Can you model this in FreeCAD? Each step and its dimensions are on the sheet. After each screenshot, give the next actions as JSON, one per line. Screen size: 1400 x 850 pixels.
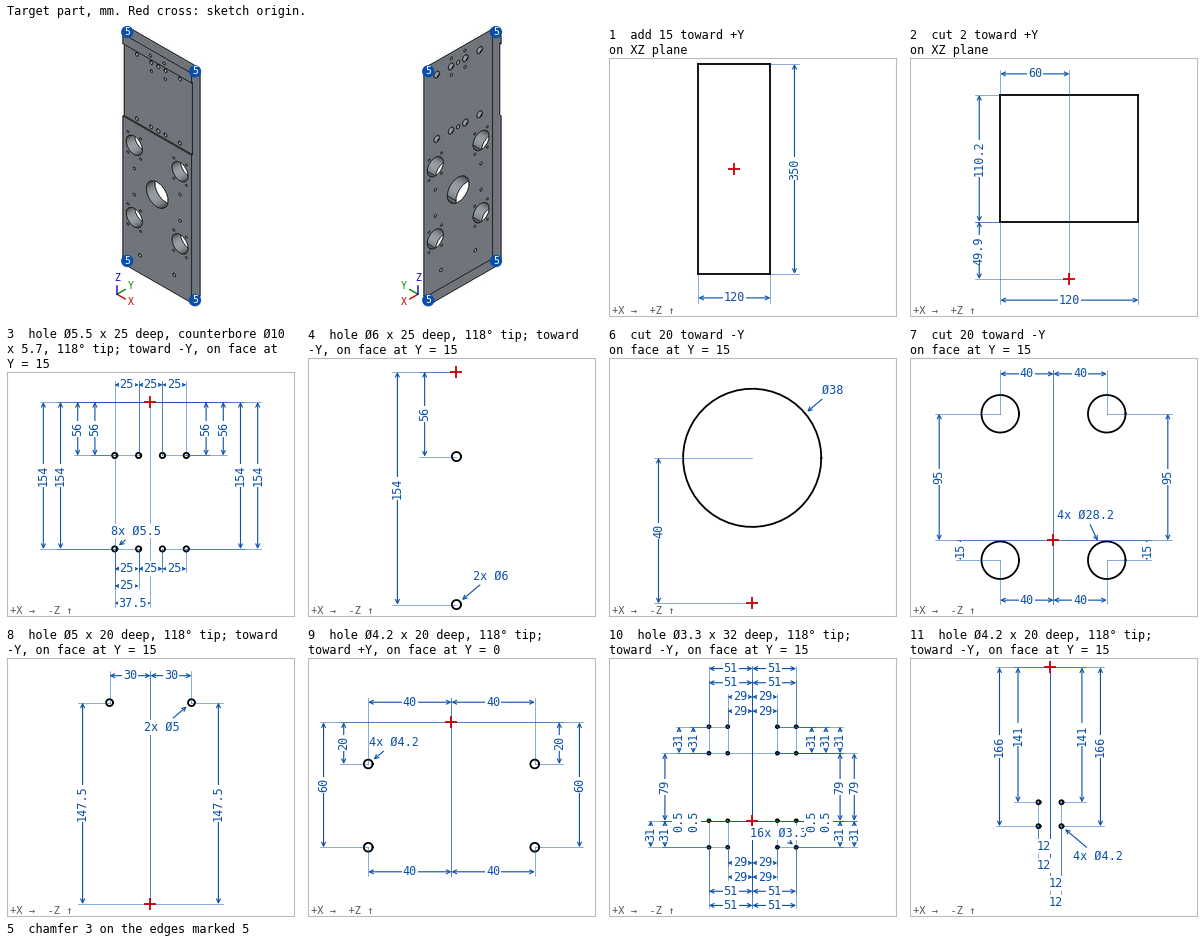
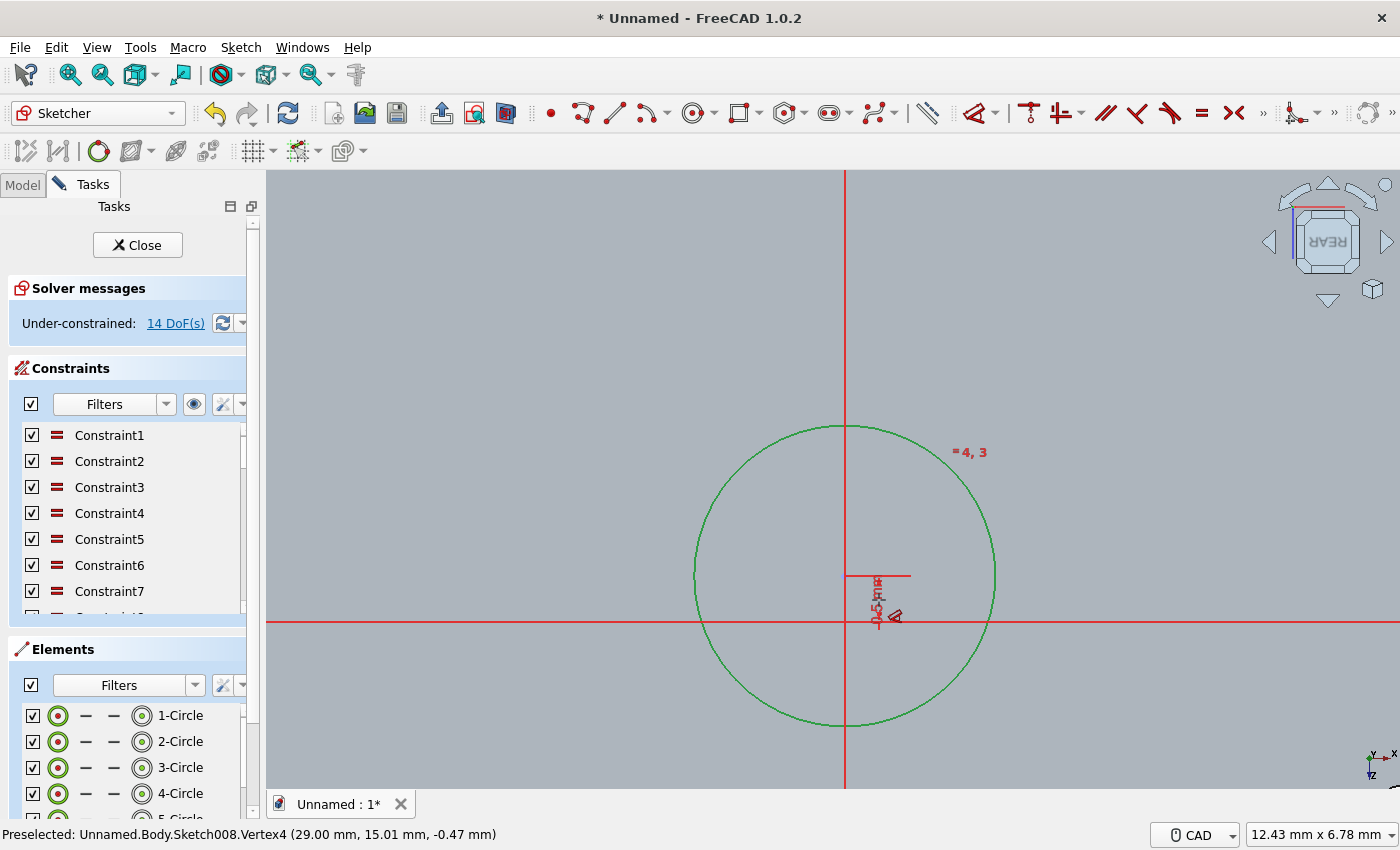
{"action": "scroll", "coordinate": [853, 601], "scroll_direction": "down", "scroll_amount": 17}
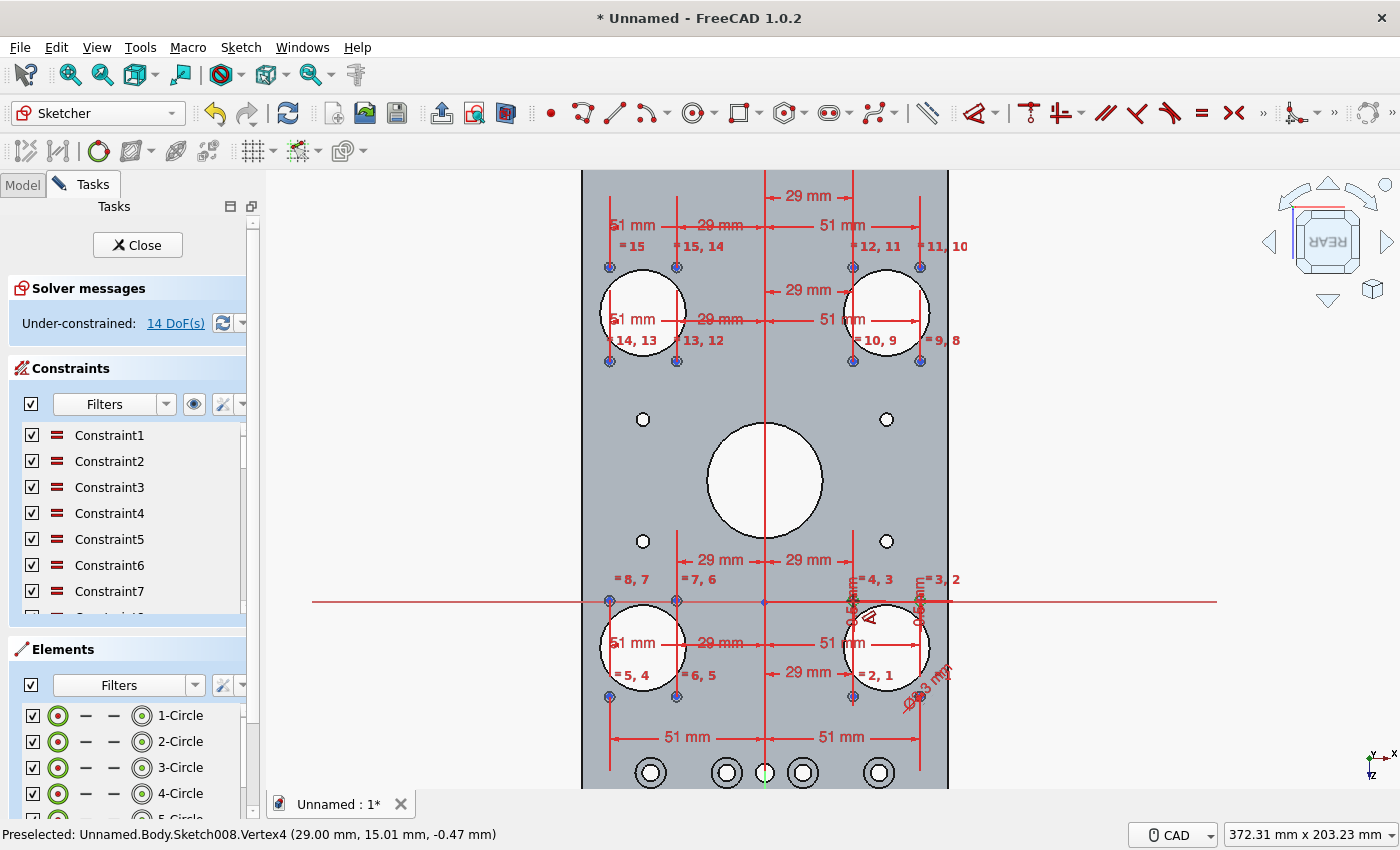
{"action": "scroll", "coordinate": [677, 601], "scroll_direction": "up", "scroll_amount": 17}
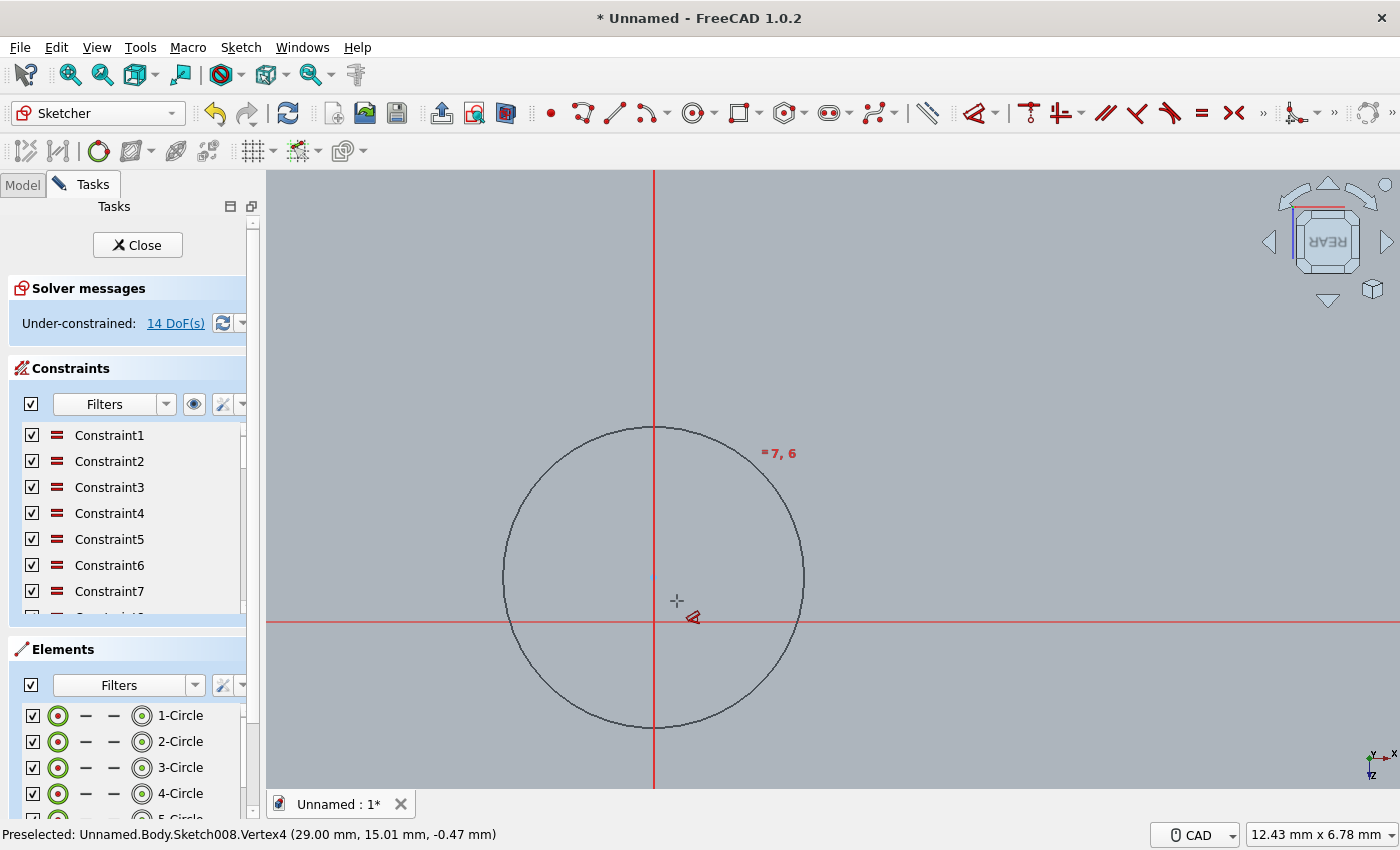
{"action": "left_click", "coordinate": [654, 577]}
{"action": "left_click", "coordinate": [620, 600]}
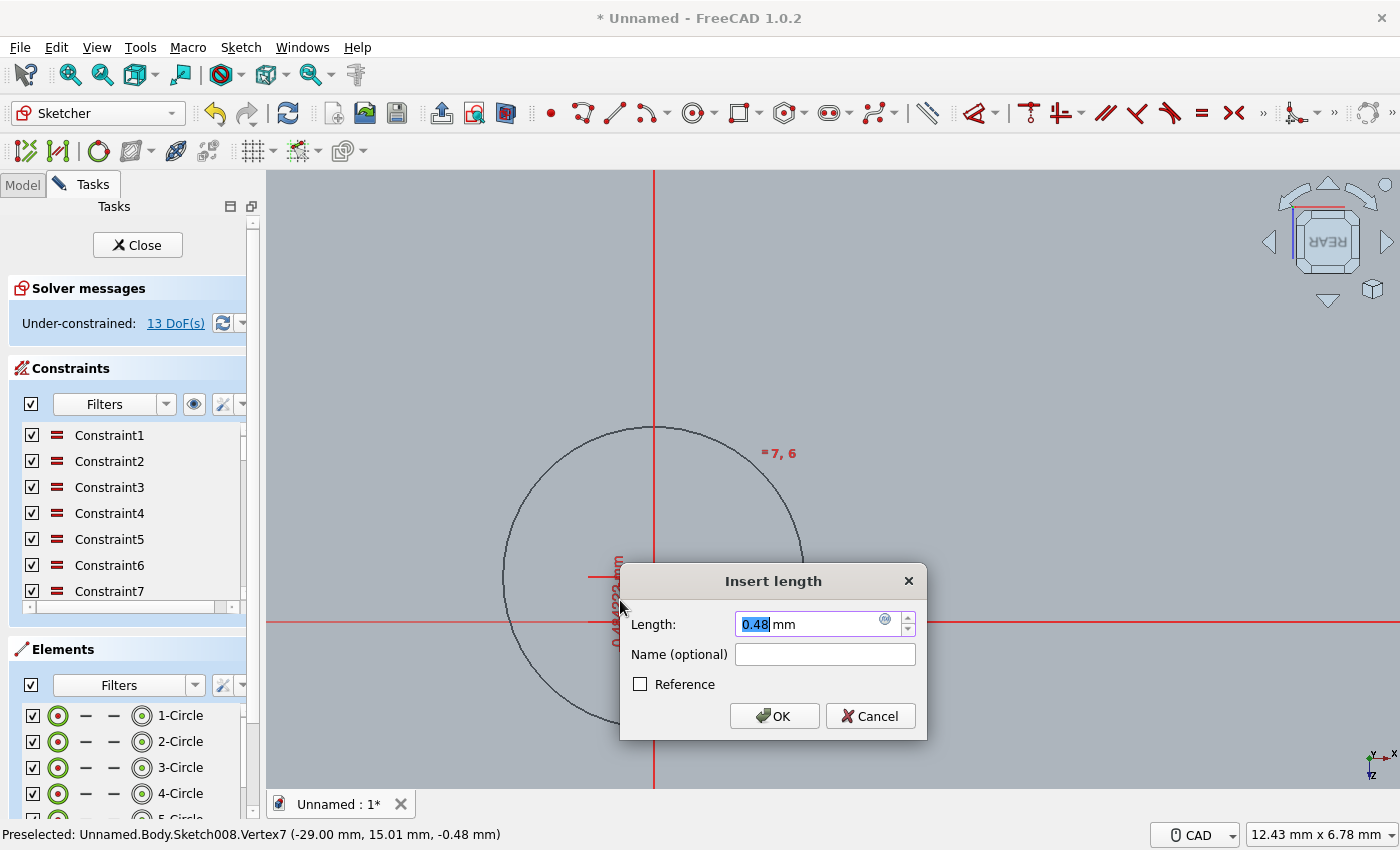
{"action": "type", "text": "0.5"}
{"action": "key", "text": "Return"}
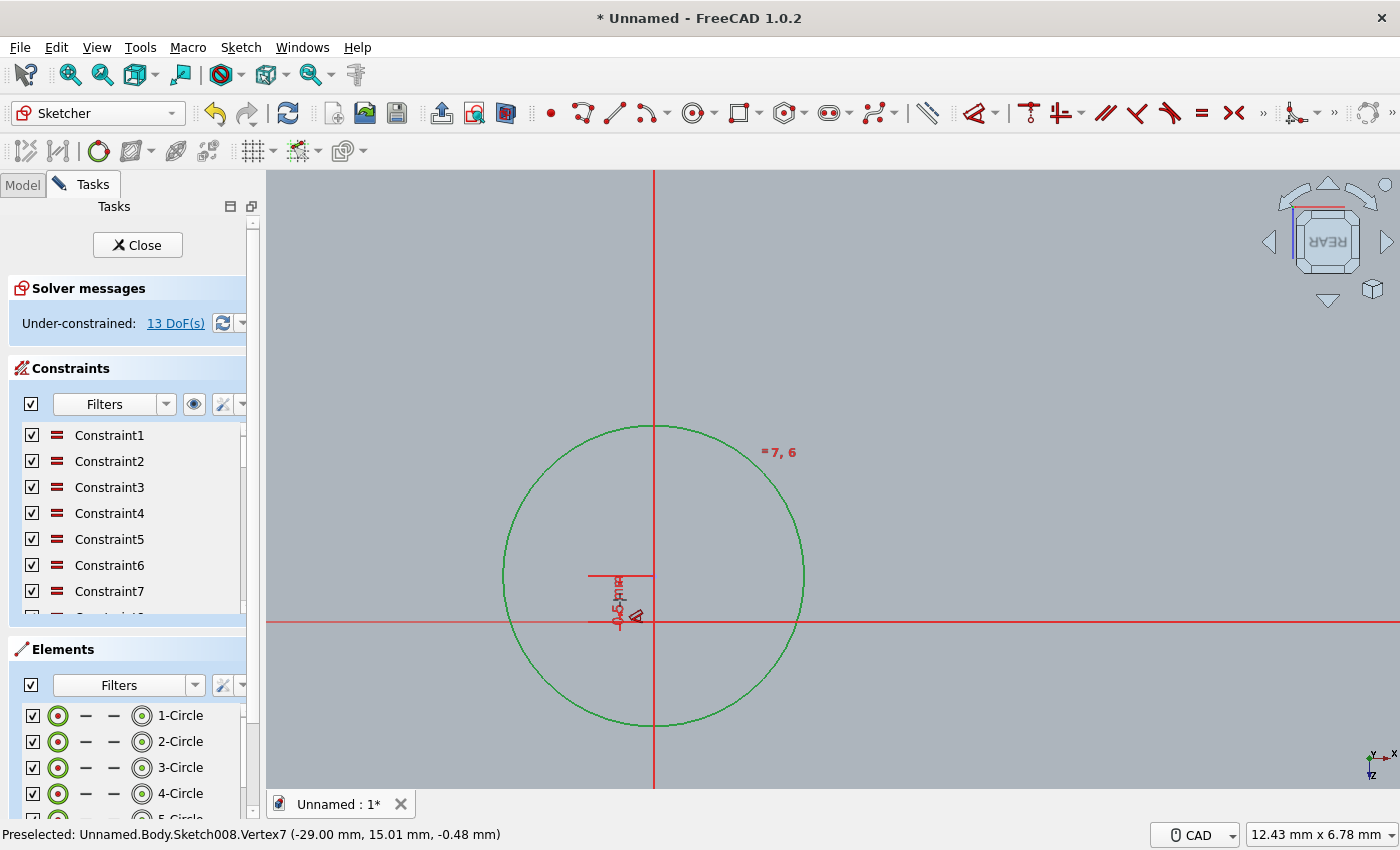
{"action": "scroll", "coordinate": [677, 601], "scroll_direction": "down", "scroll_amount": 17}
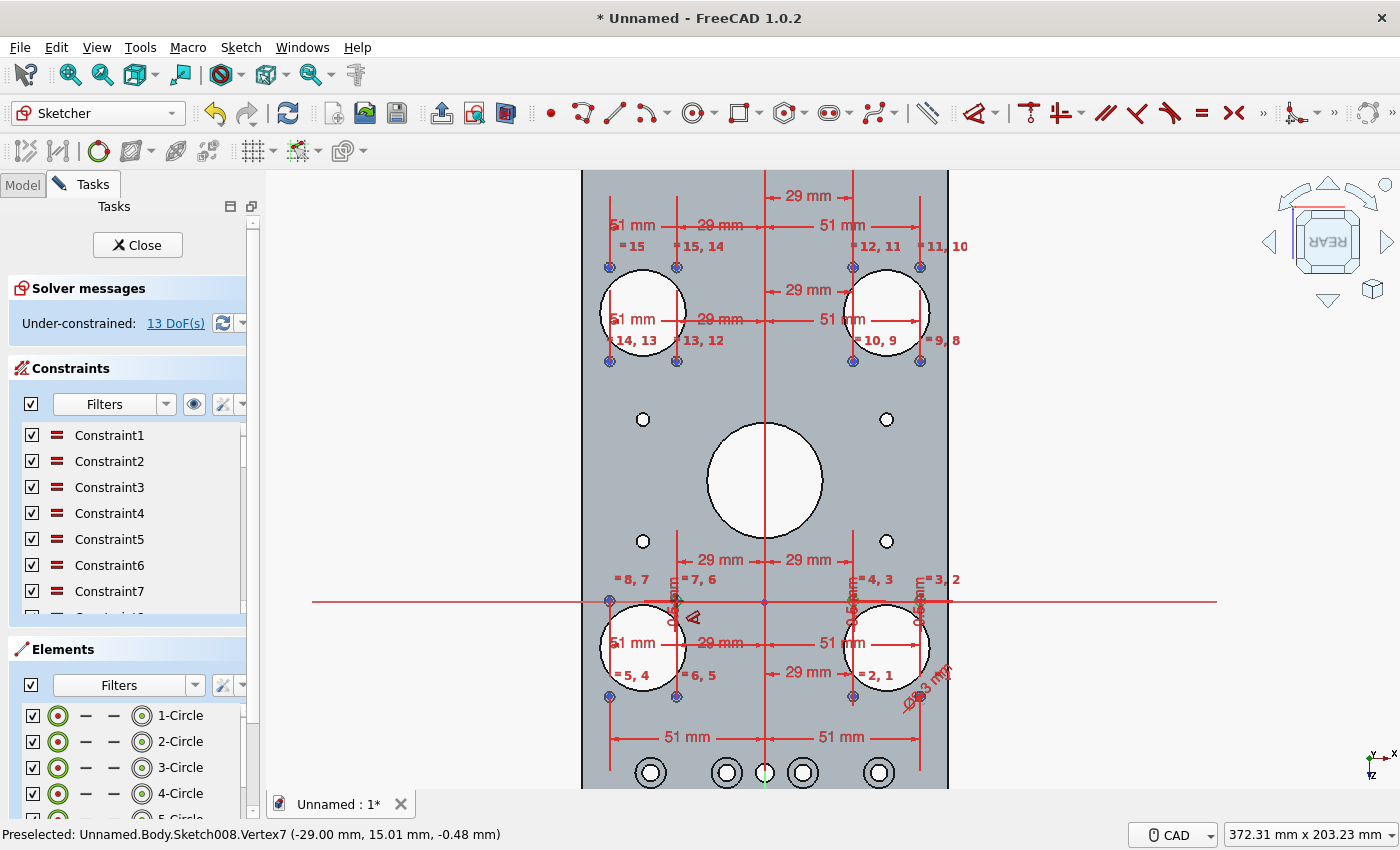
{"action": "scroll", "coordinate": [610, 601], "scroll_direction": "up", "scroll_amount": 17}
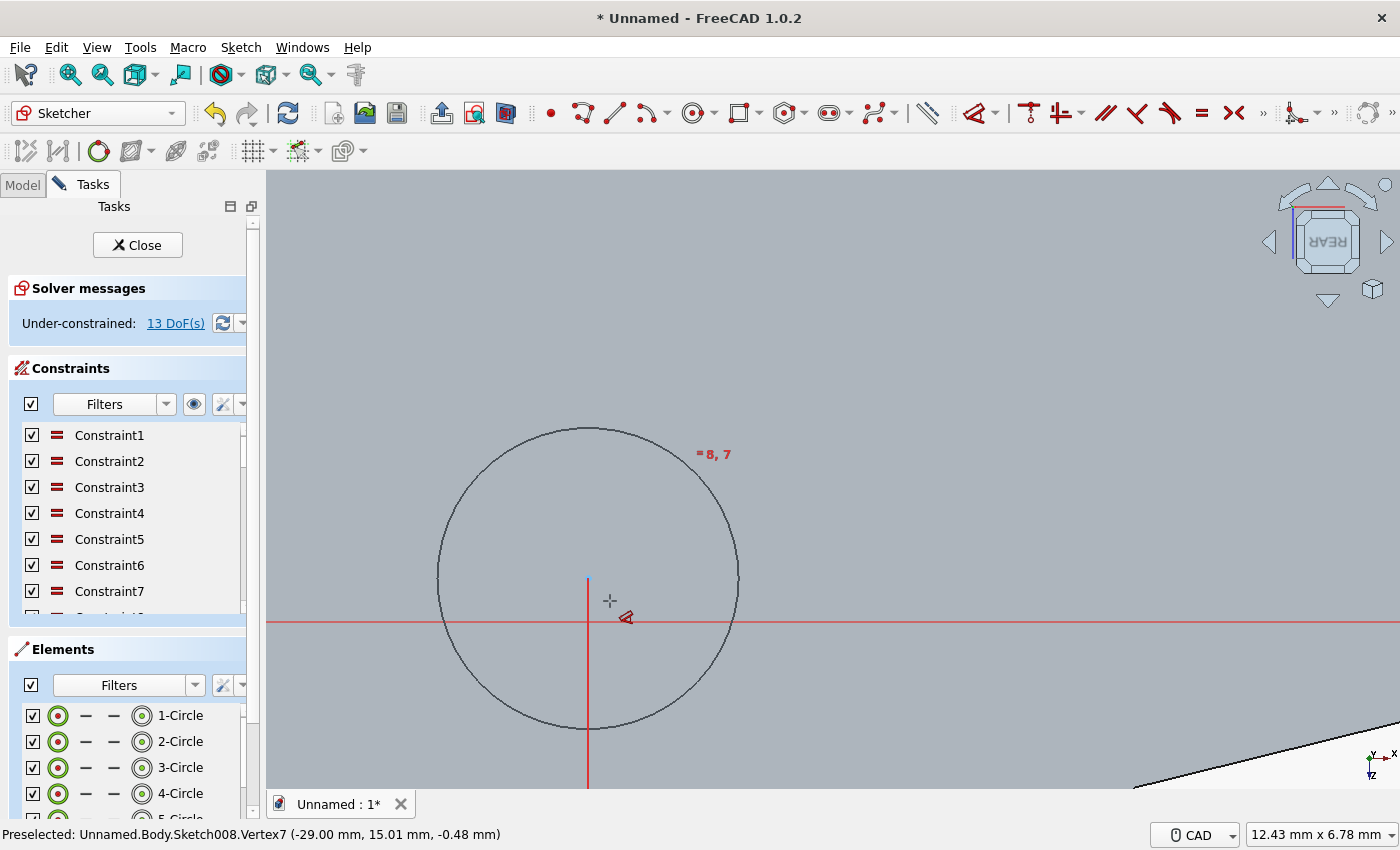
{"action": "left_click", "coordinate": [588, 579]}
{"action": "left_click", "coordinate": [554, 600]}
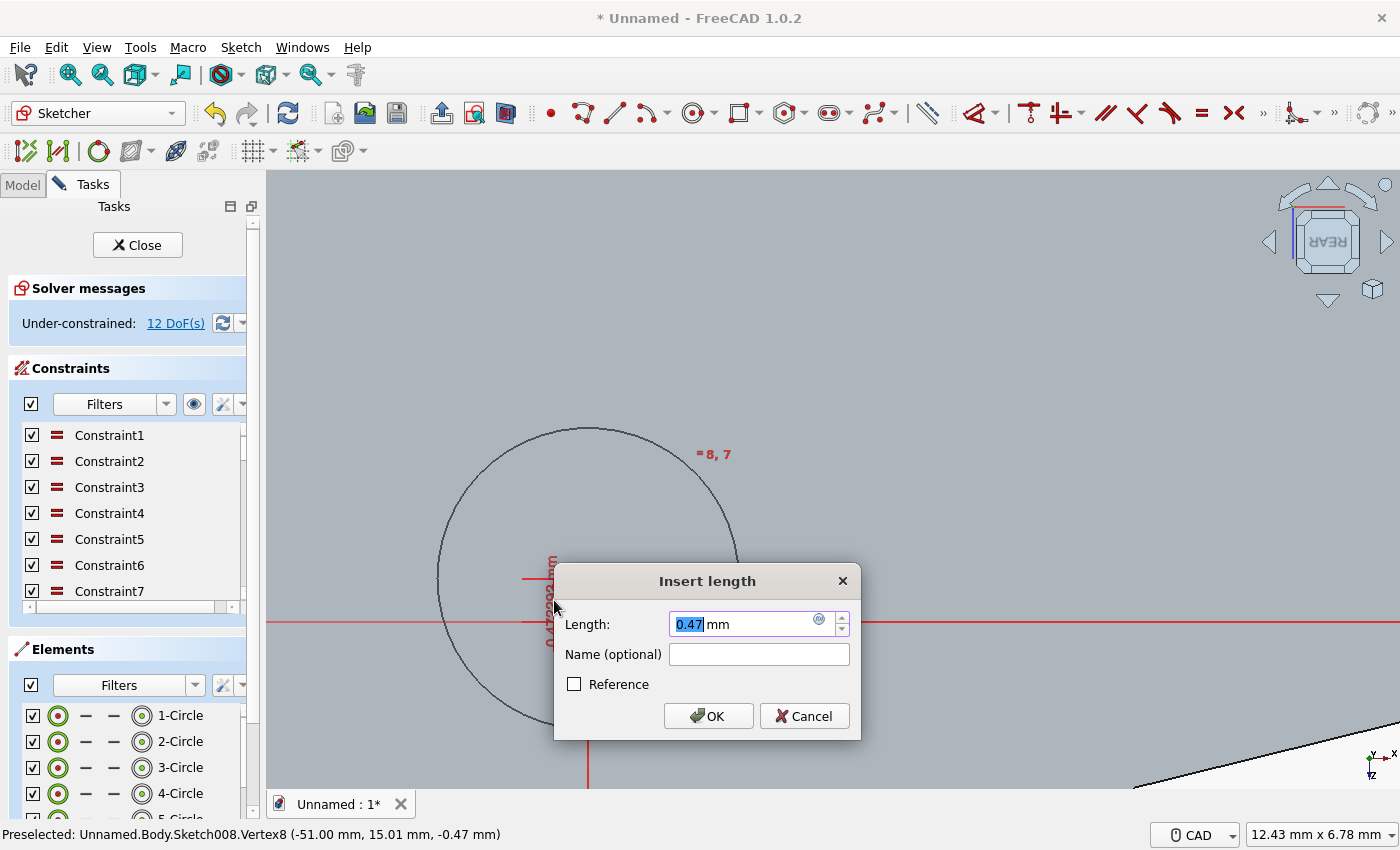
{"action": "type", "text": "0.5"}
{"action": "key", "text": "Return"}